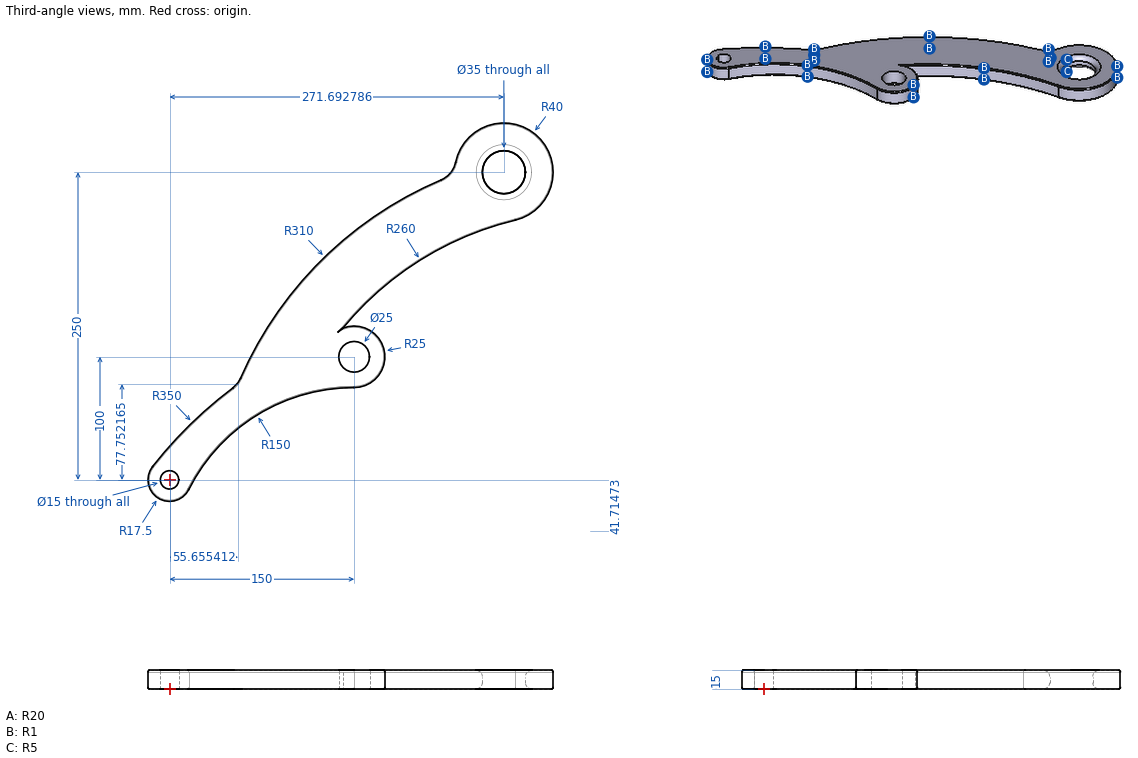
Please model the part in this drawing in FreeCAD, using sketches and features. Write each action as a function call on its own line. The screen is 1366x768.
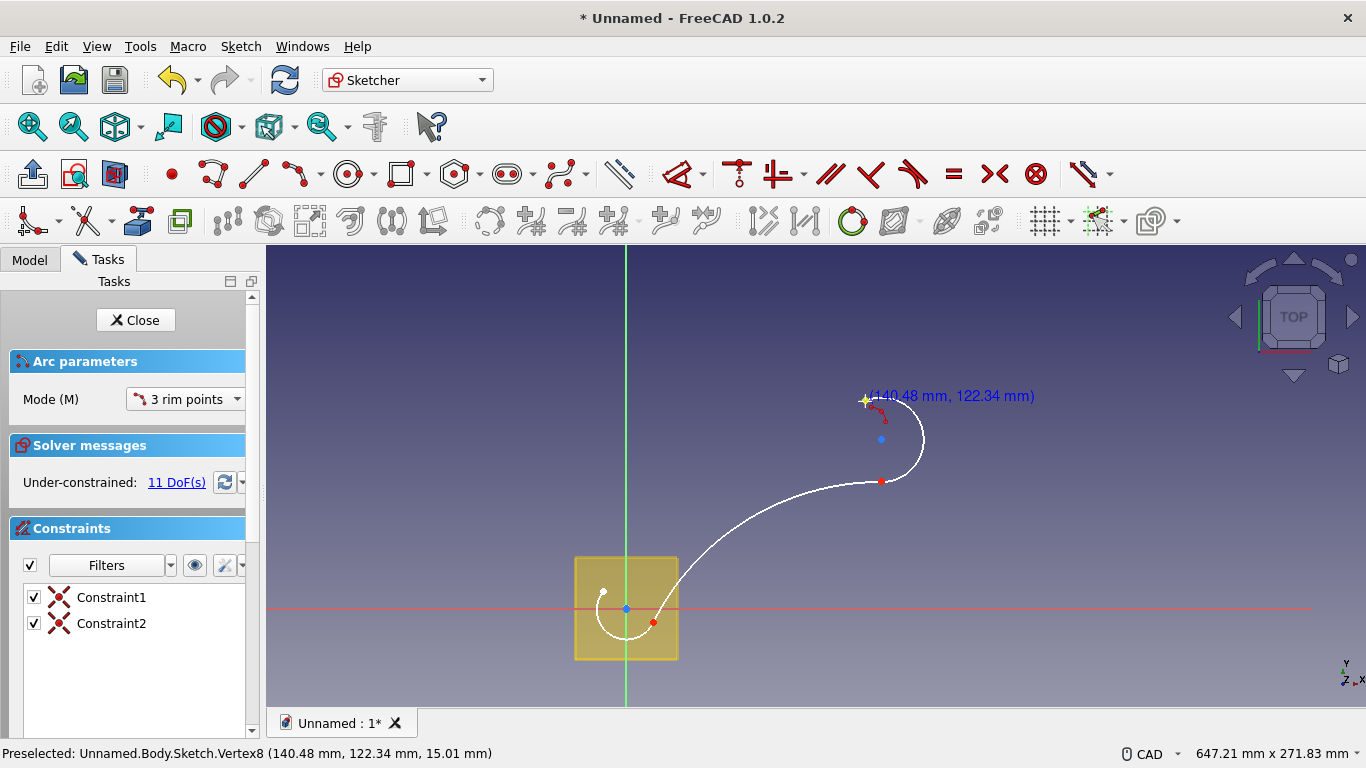
scroll(604, 591, down, 3)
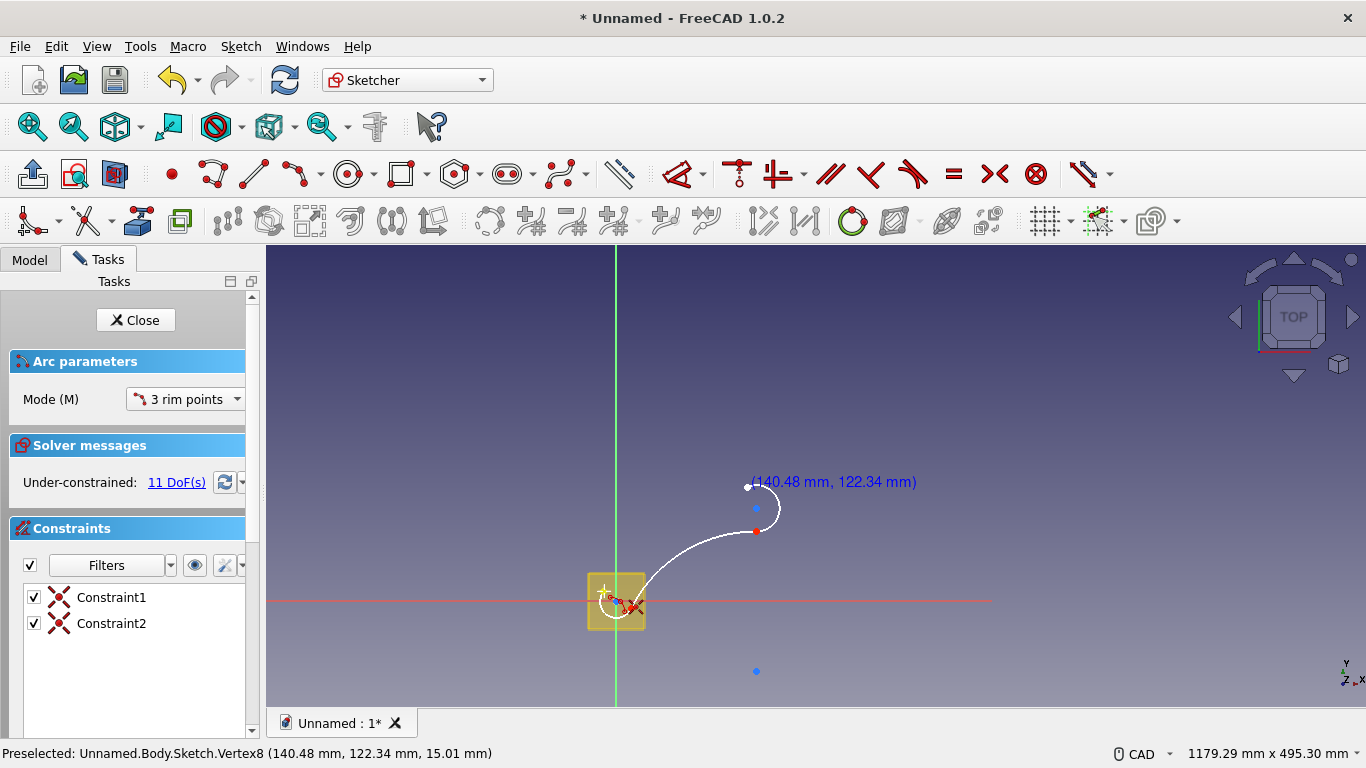
click(878, 404)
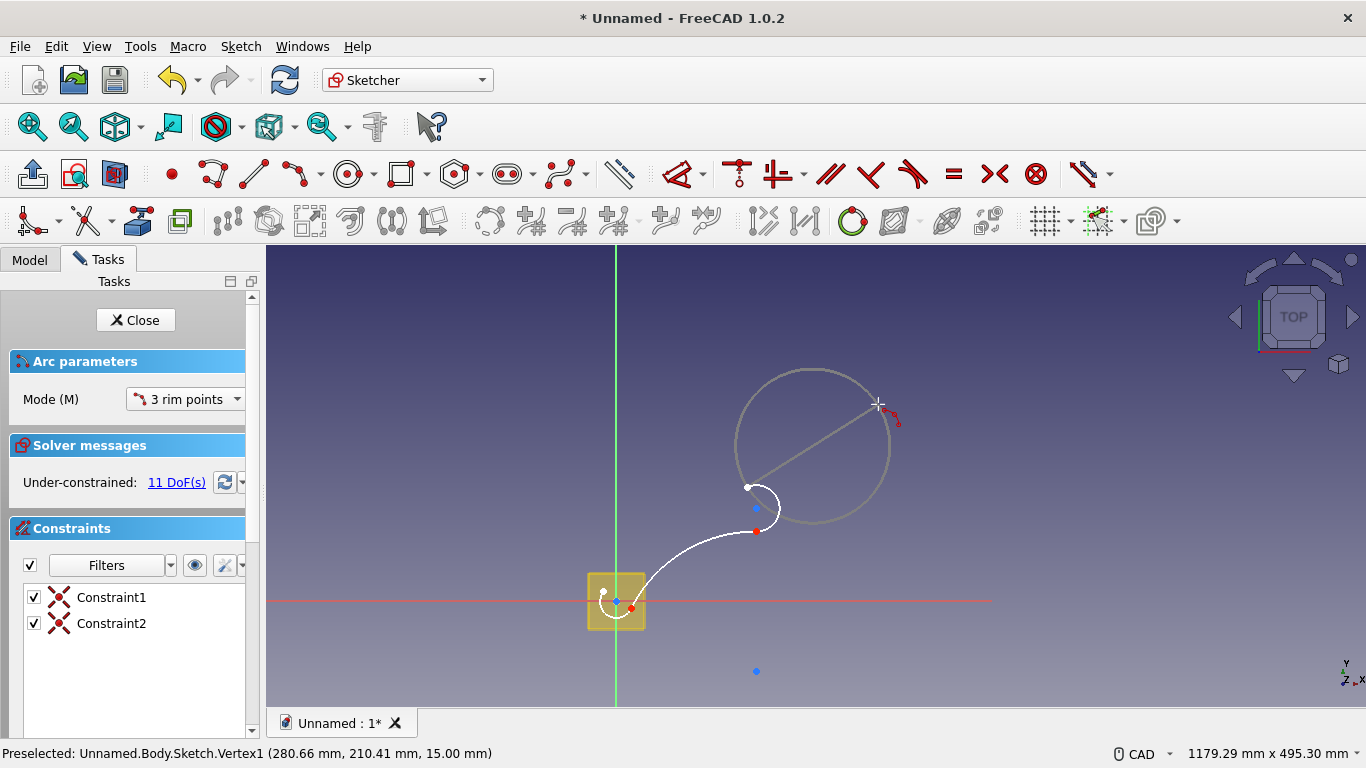
scroll(806, 435, up, 2)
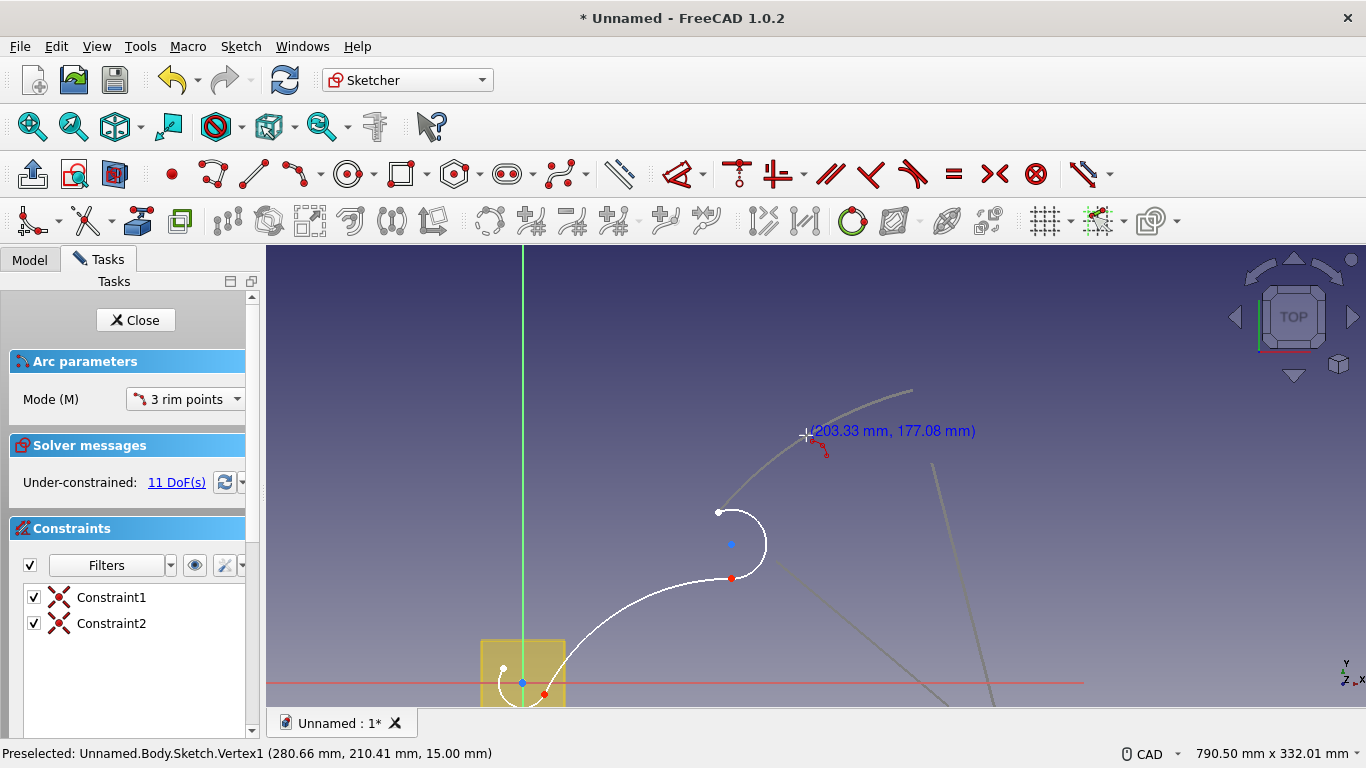
click(806, 434)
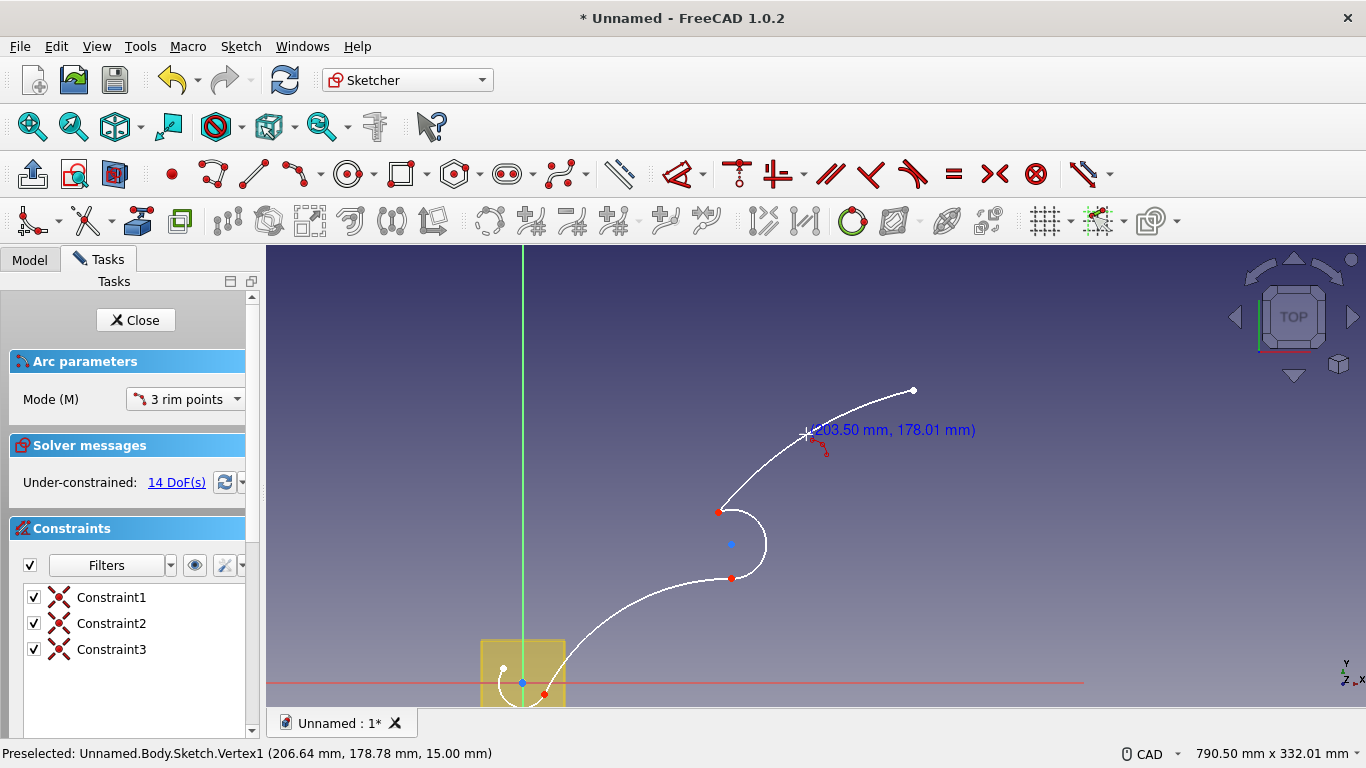
click(913, 390)
click(845, 337)
click(934, 290)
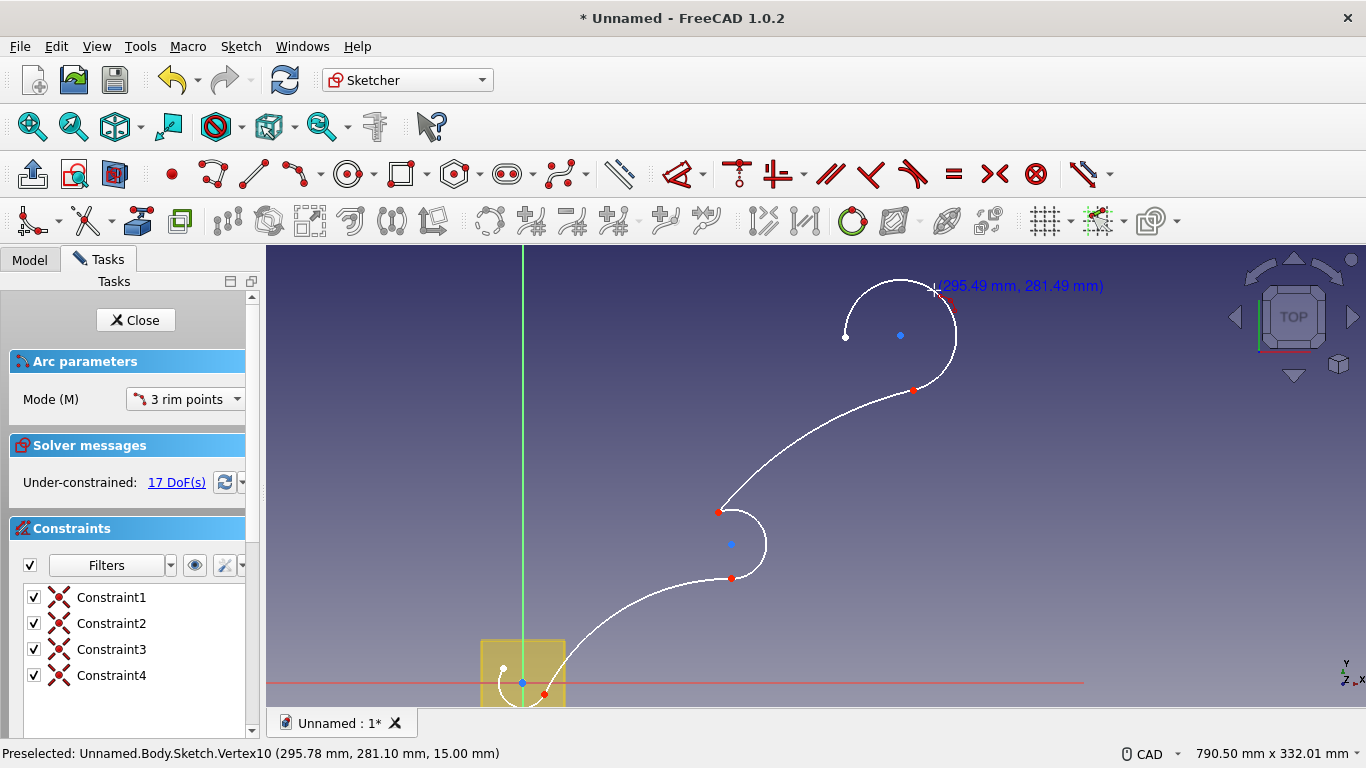
click(845, 338)
click(600, 575)
click(698, 431)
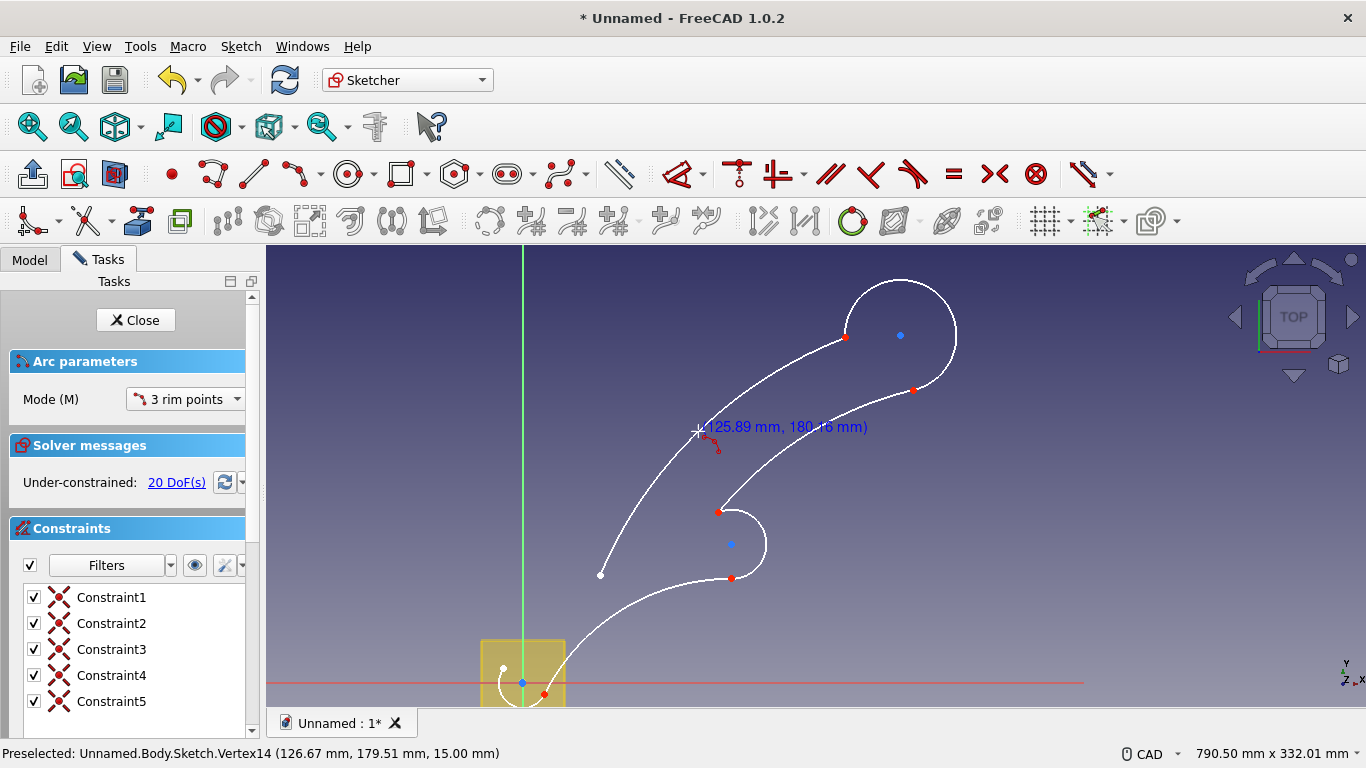
click(600, 576)
click(504, 669)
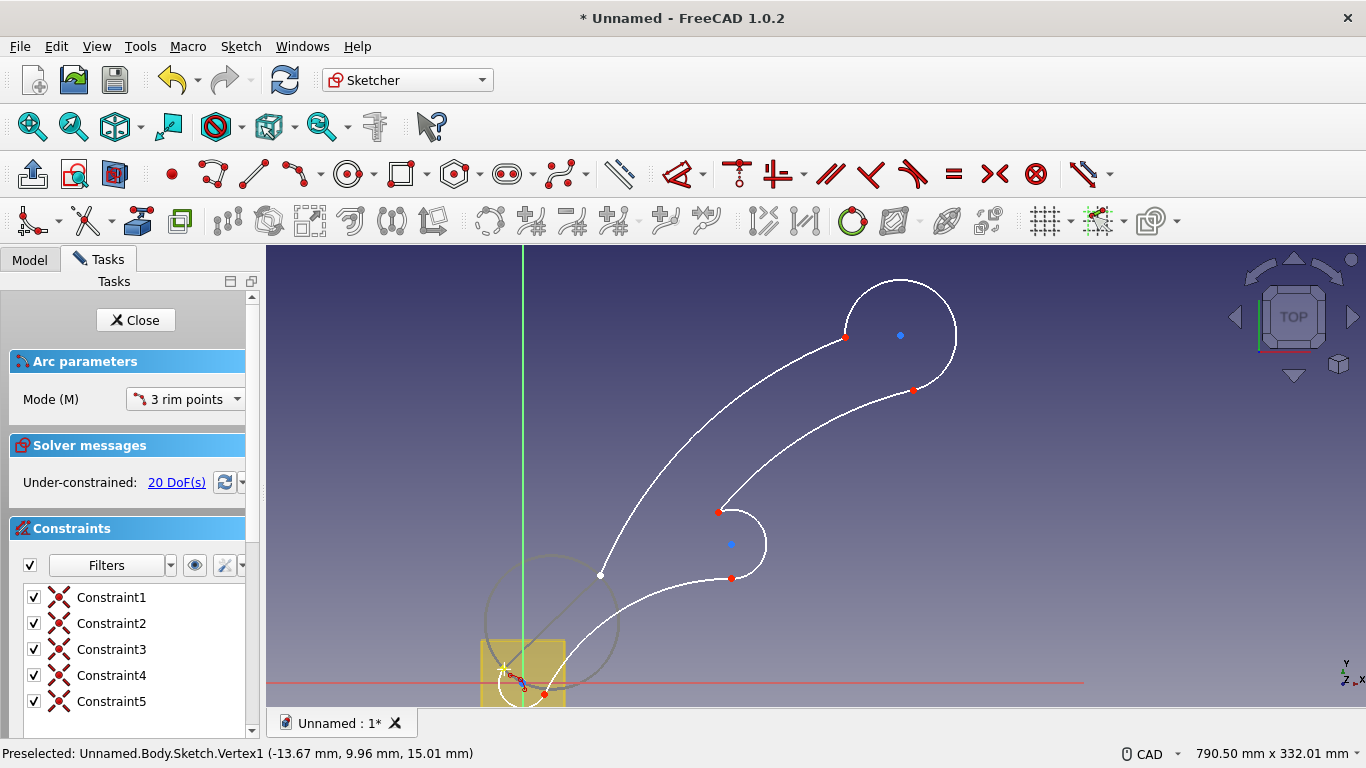
scroll(549, 618, up, 7)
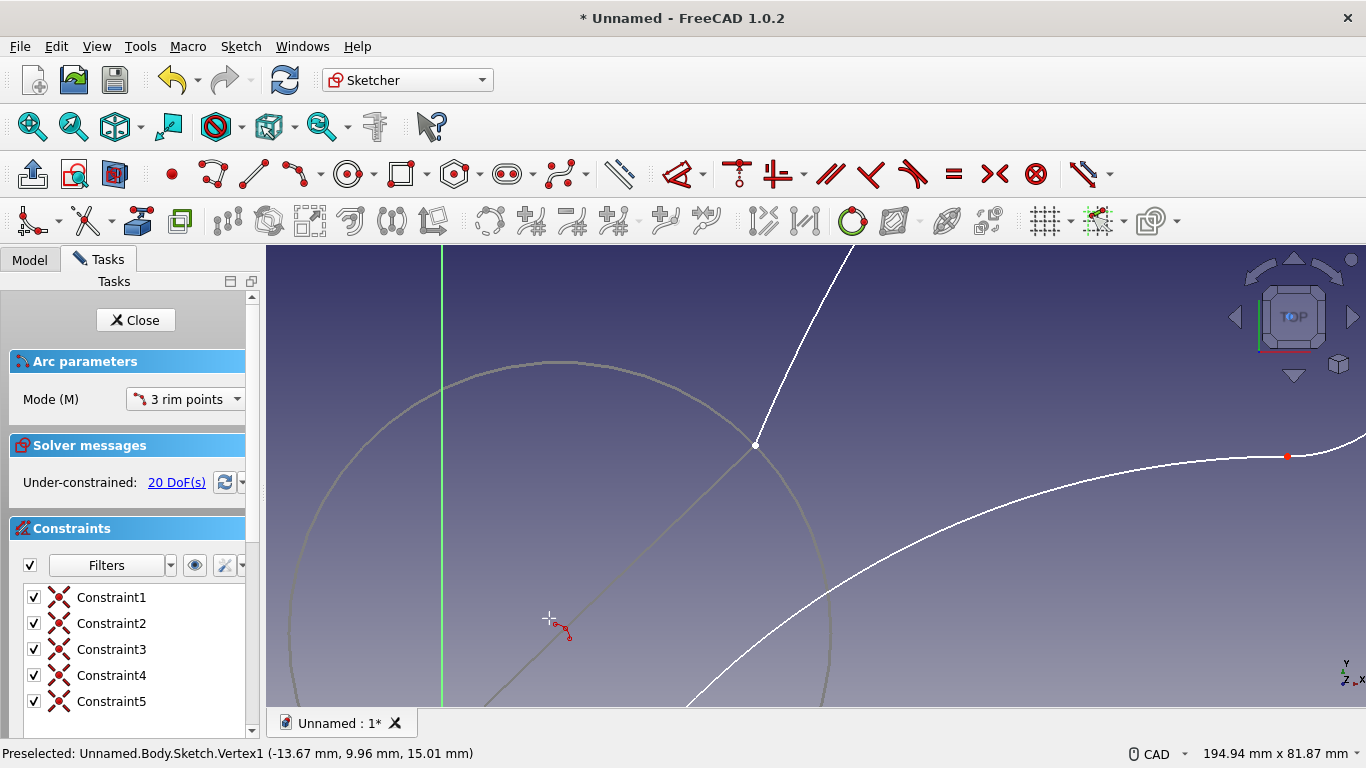
click(547, 614)
key(Escape)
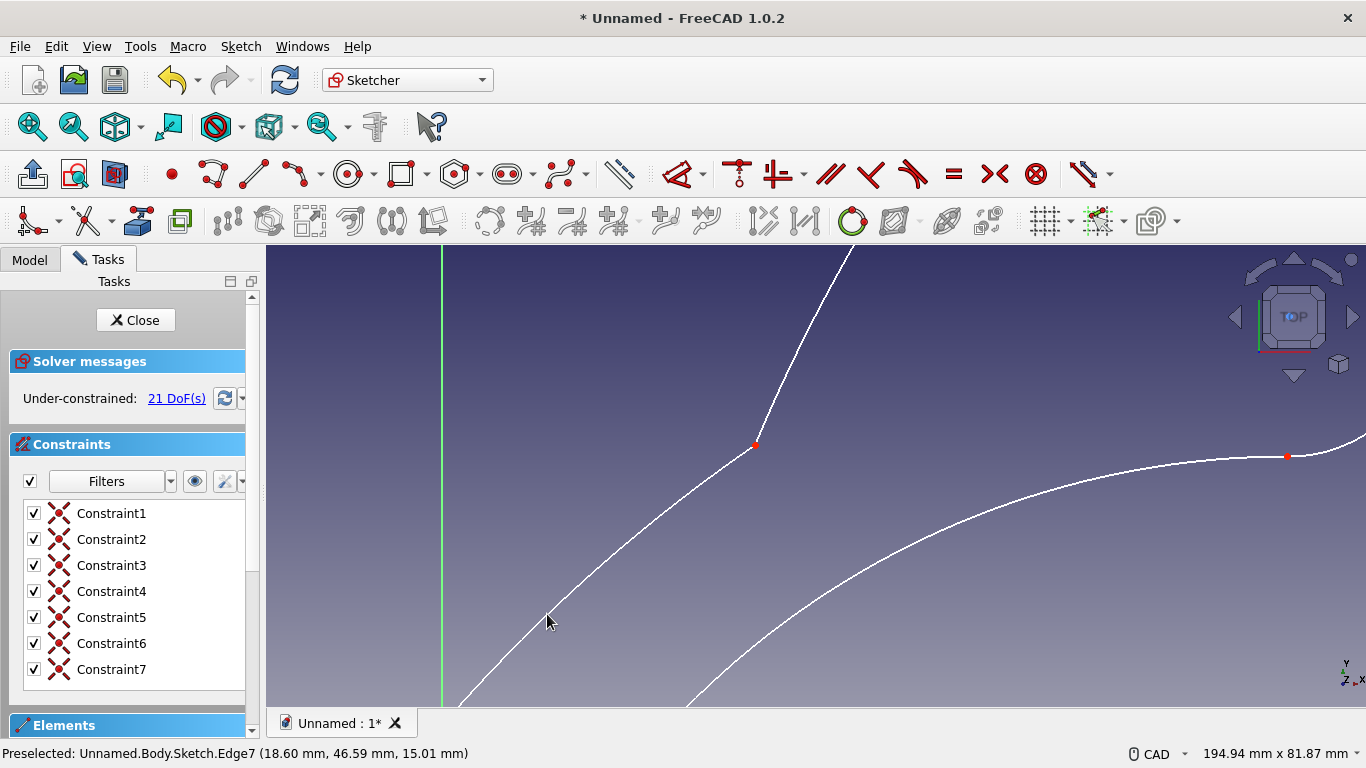
scroll(650, 546, down, 9)